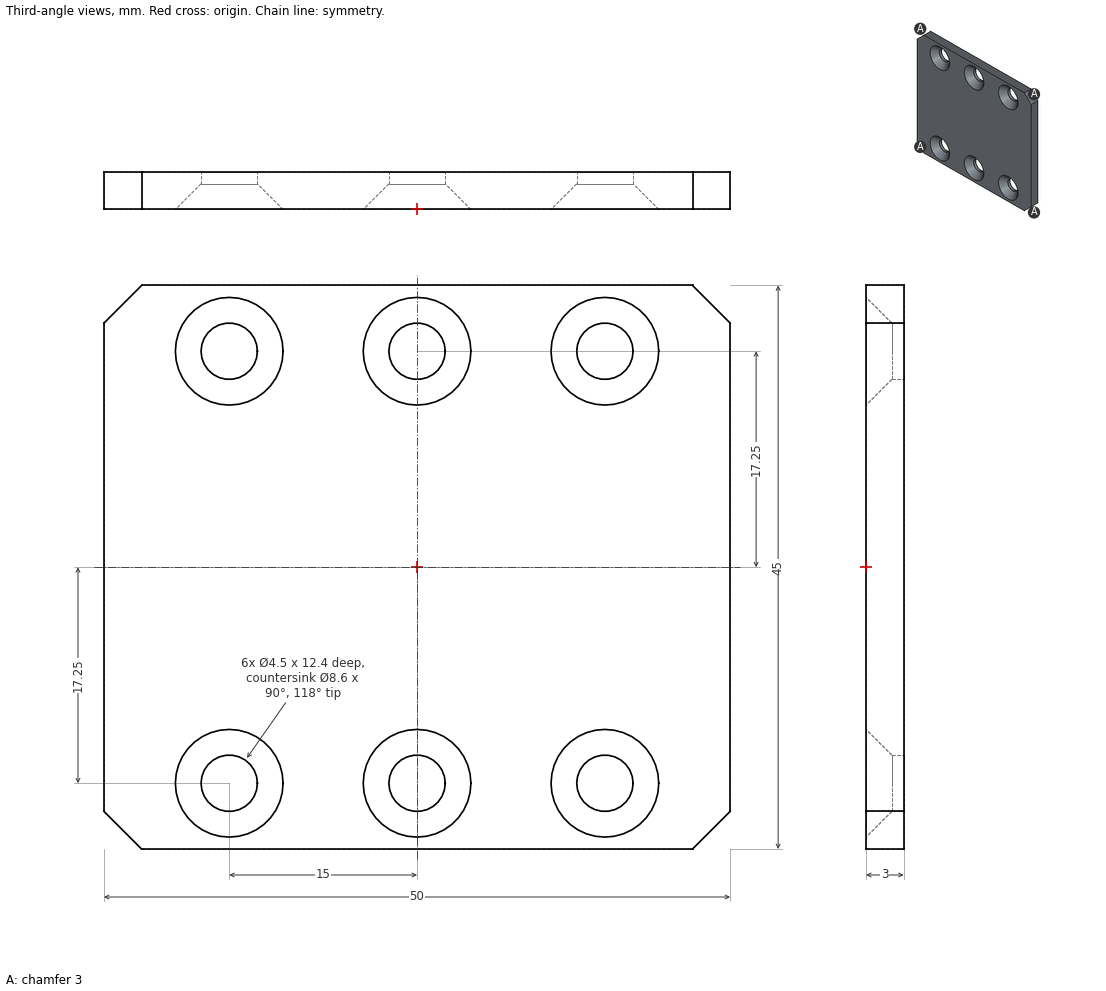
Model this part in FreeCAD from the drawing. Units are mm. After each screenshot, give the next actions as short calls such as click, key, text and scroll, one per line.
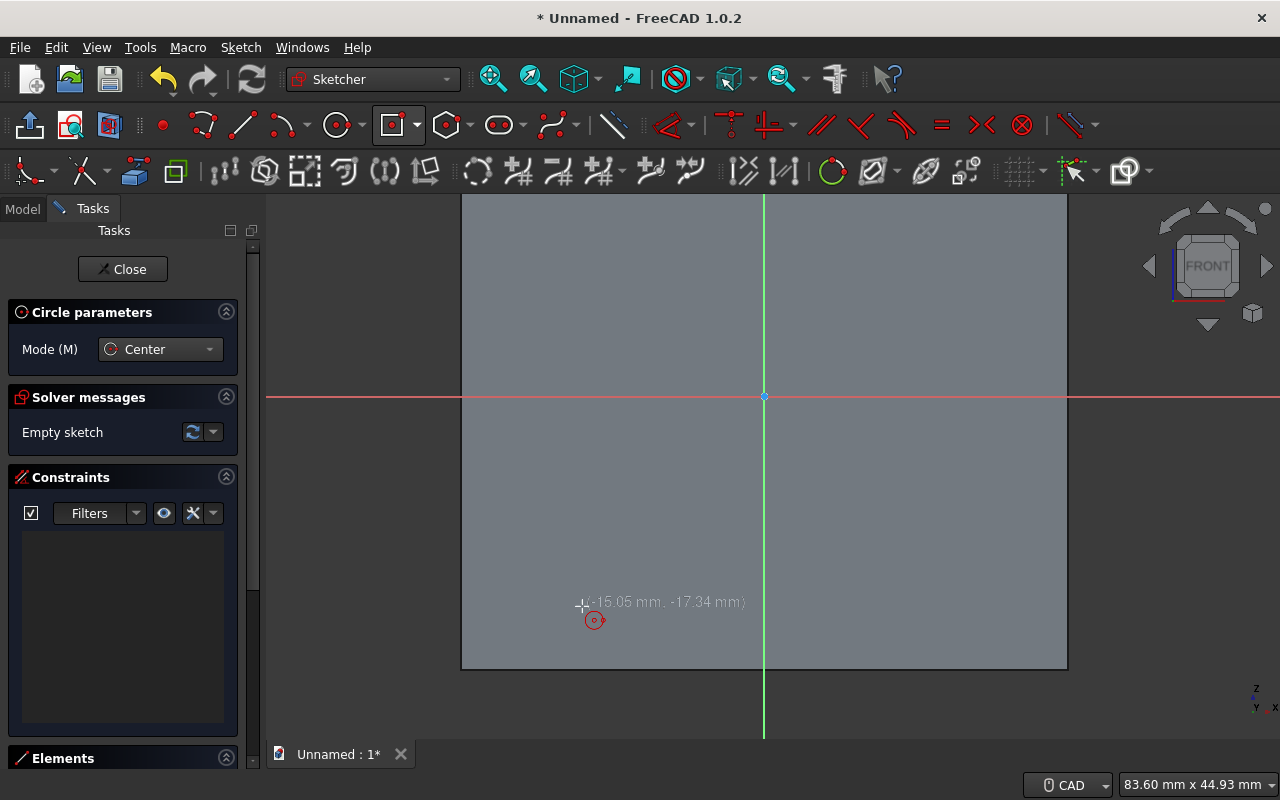
click(582, 606)
move(602, 587)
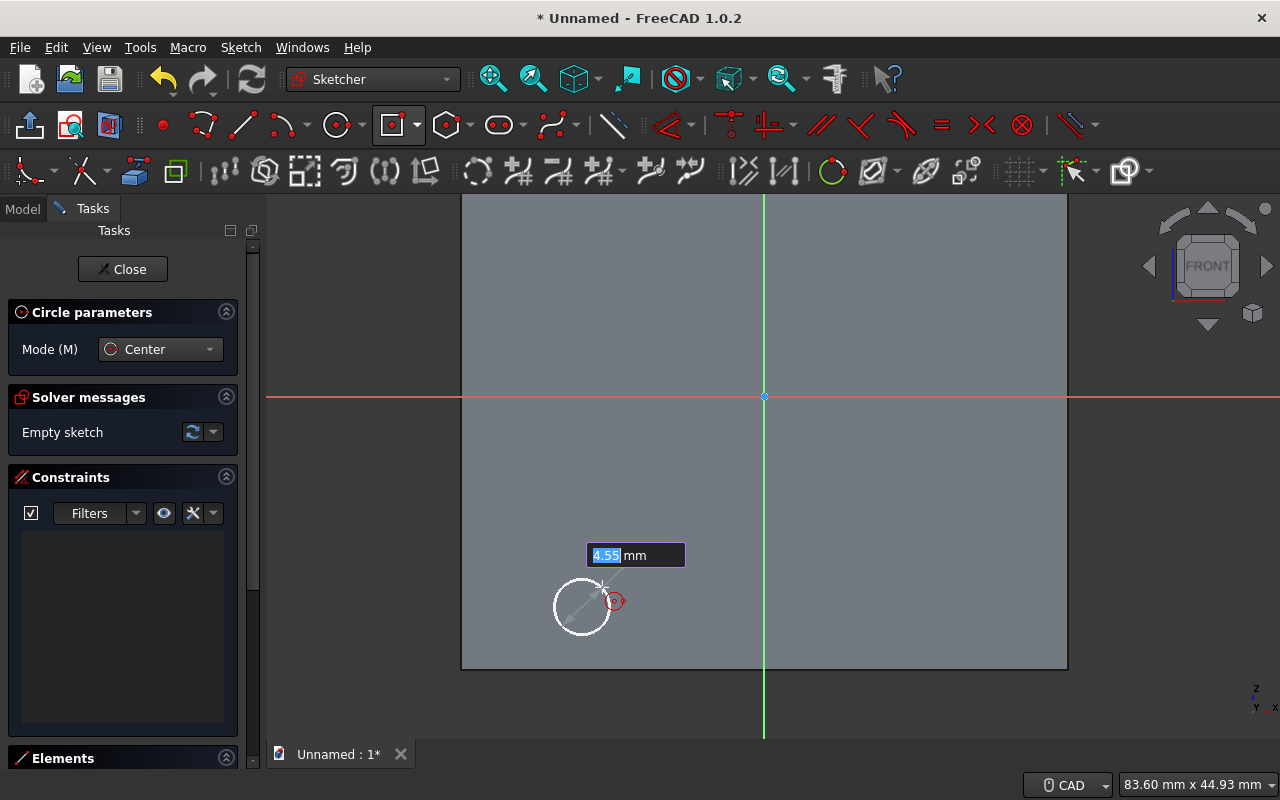
text(4.5)
key(Return)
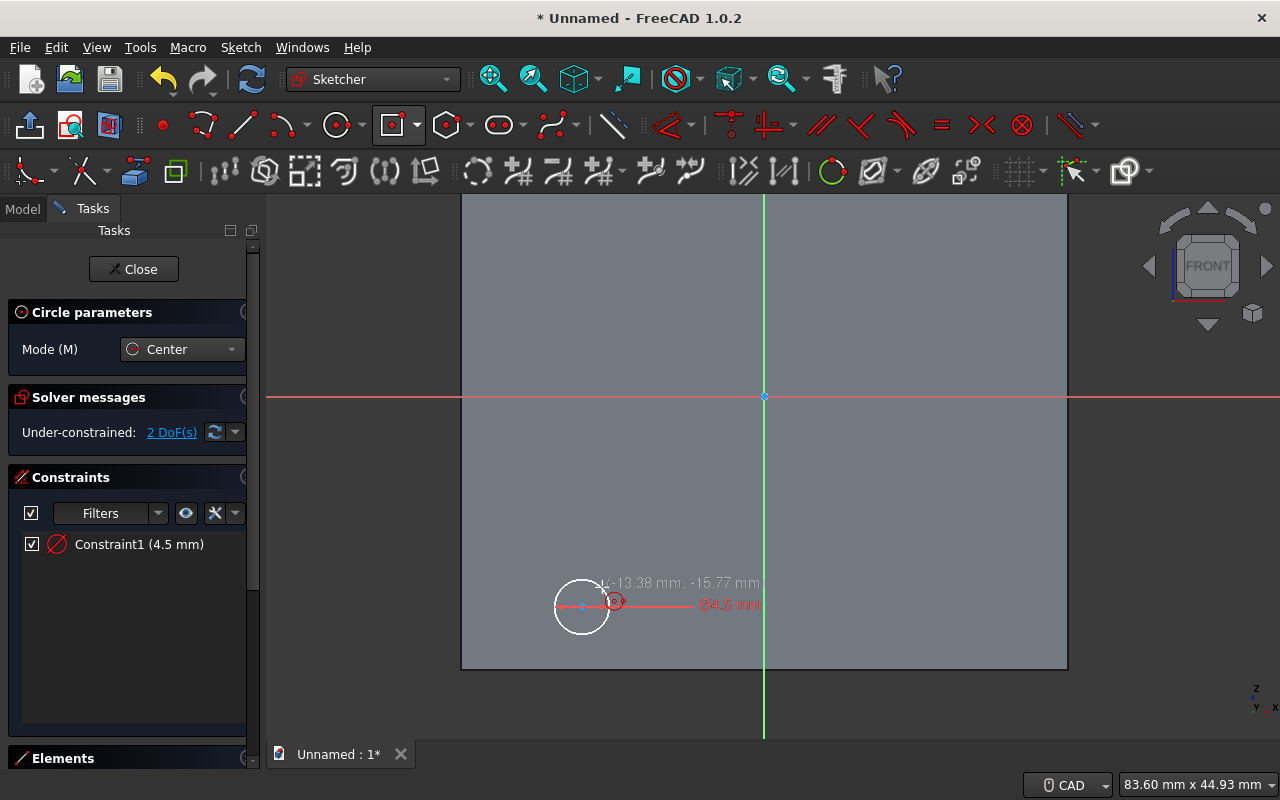
click(764, 606)
move(784, 587)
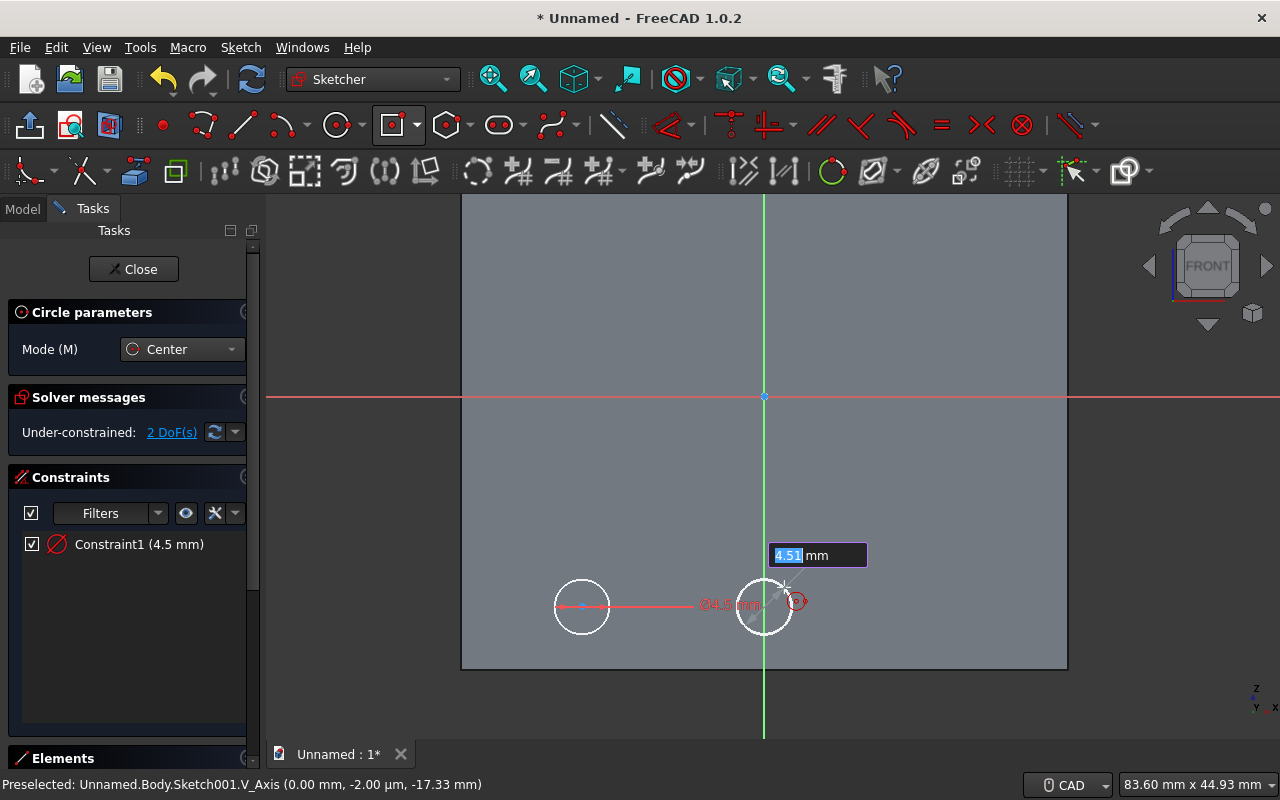
text(4.5)
key(Return)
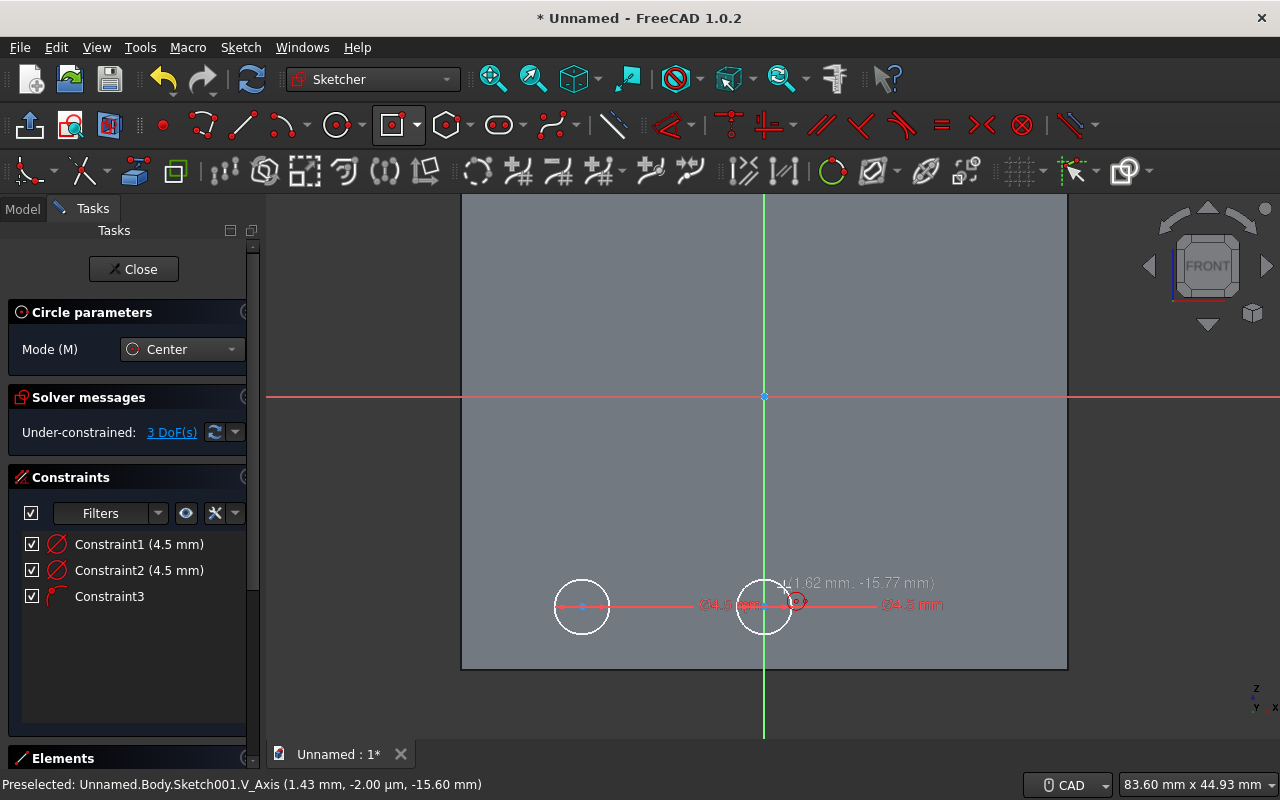
click(946, 606)
move(966, 587)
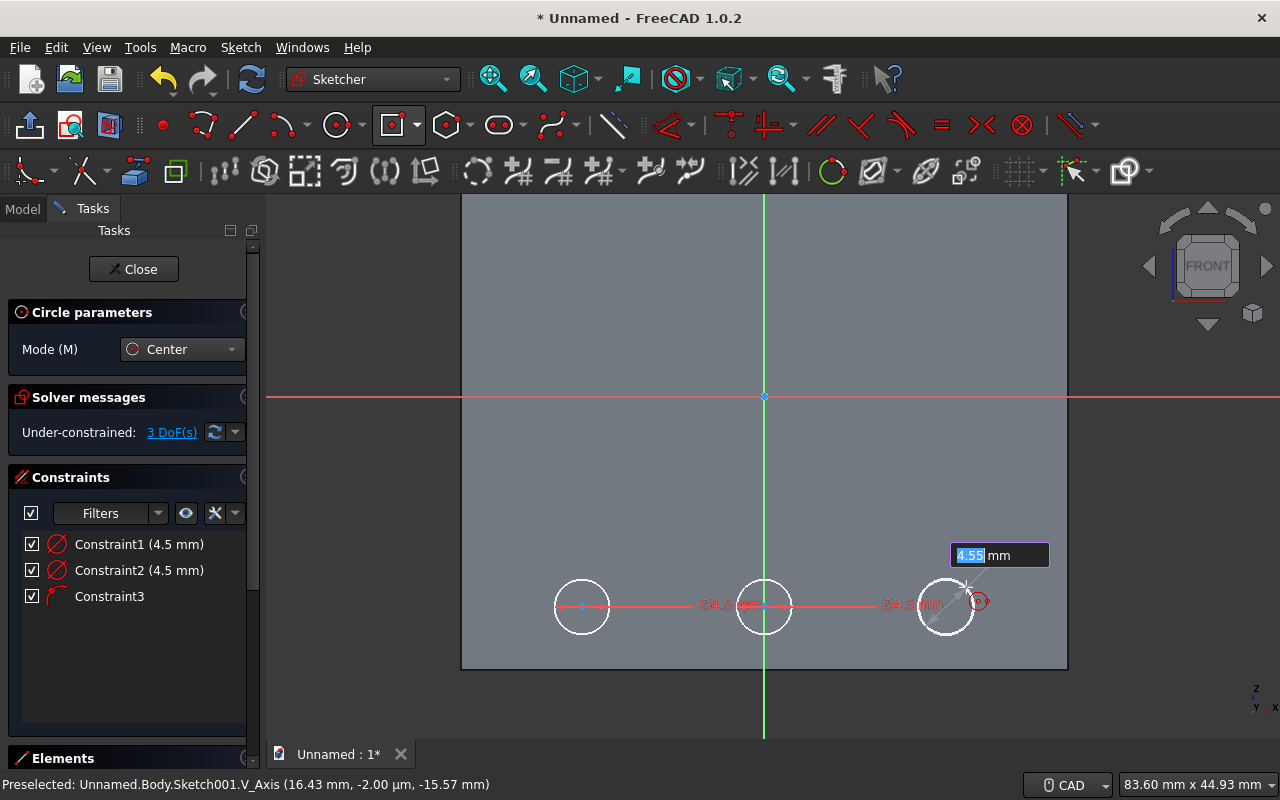
text(4.5)
key(Return)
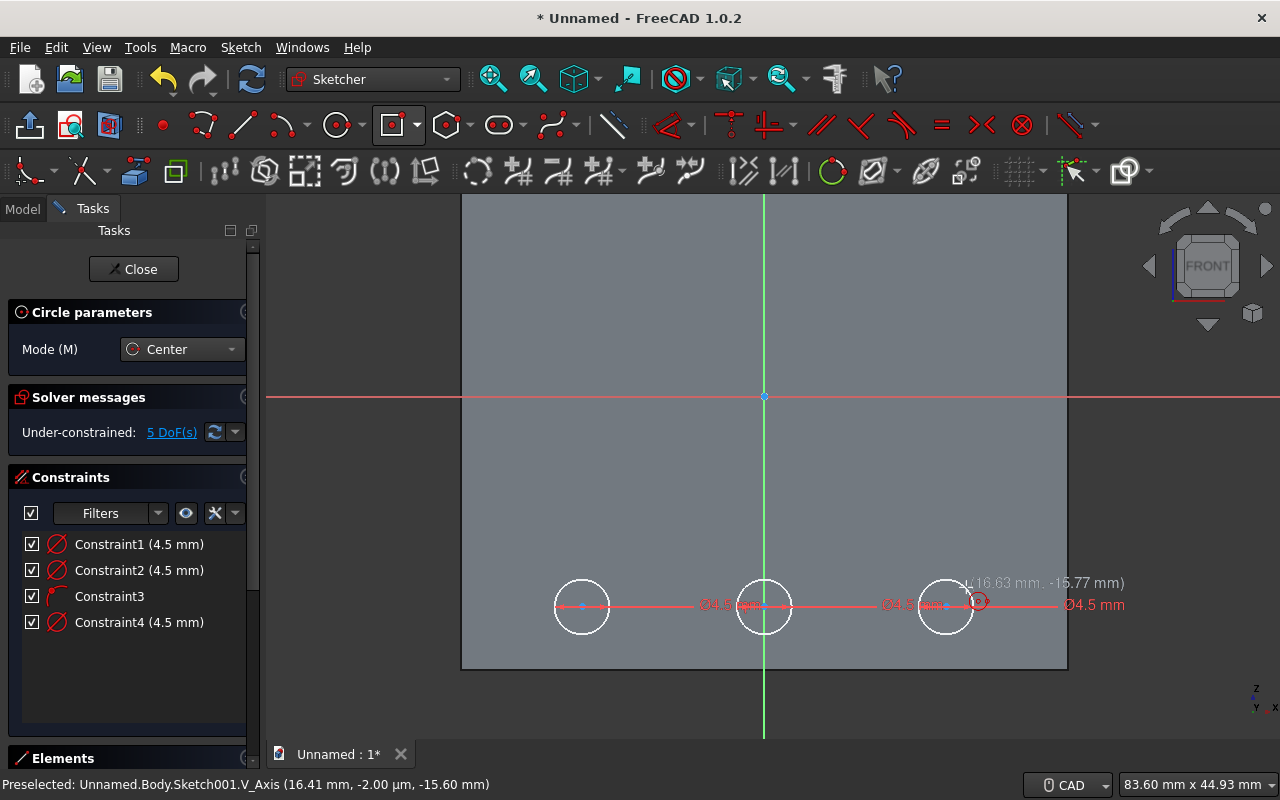
scroll(583, 608, down, 2)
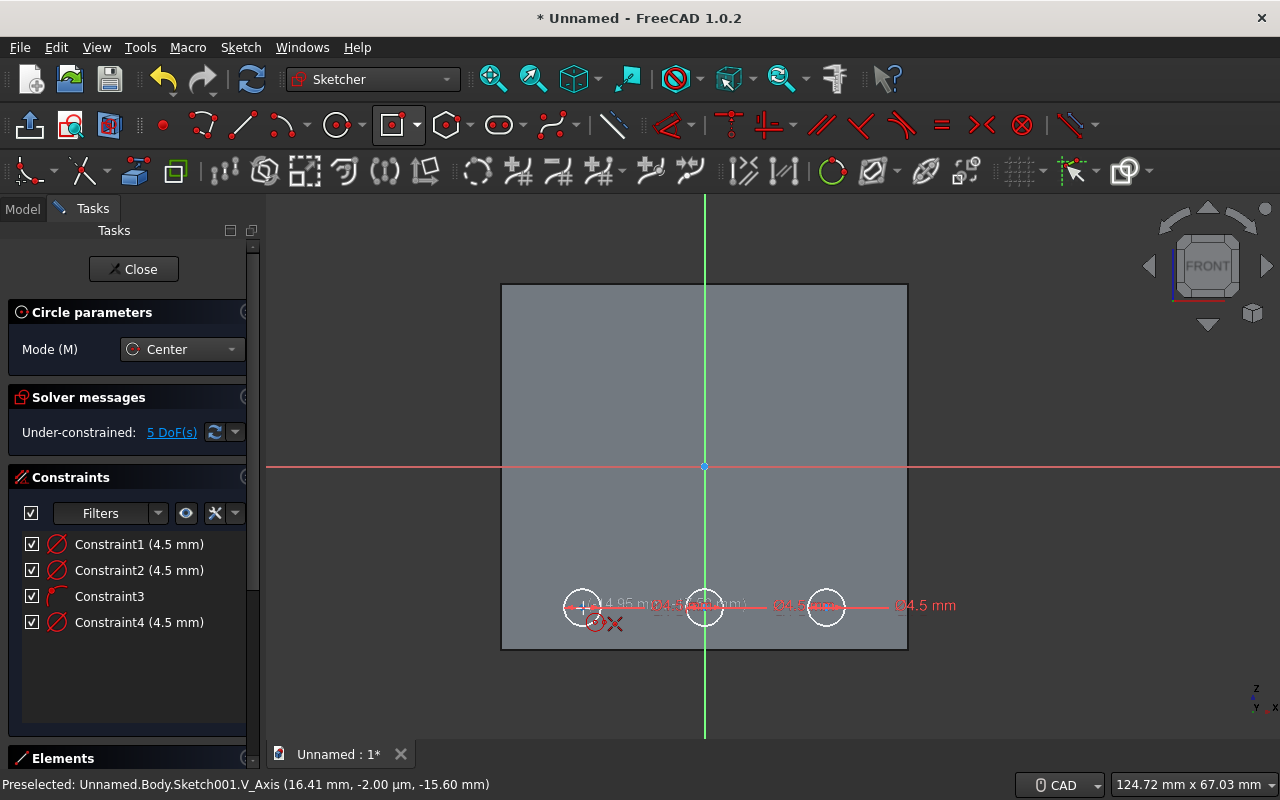
scroll(827, 326, up, 2)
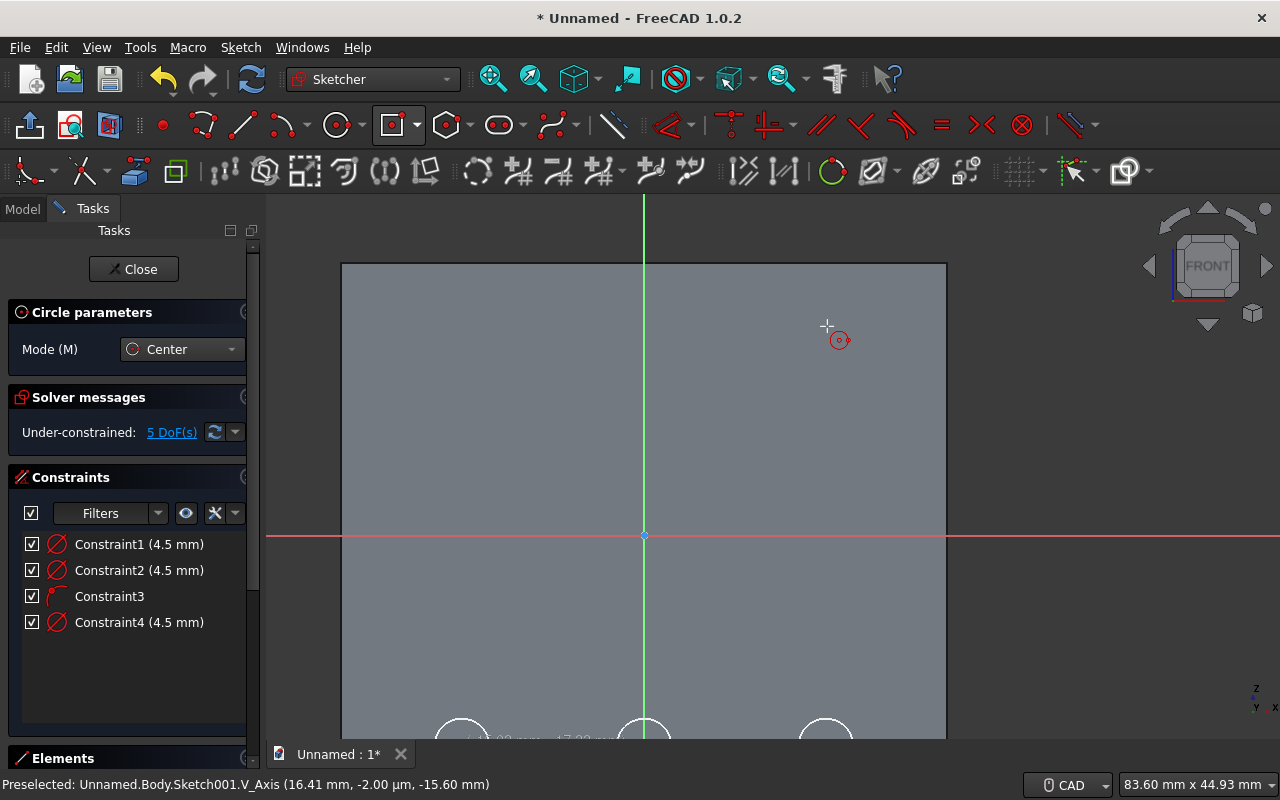
click(826, 327)
move(845, 307)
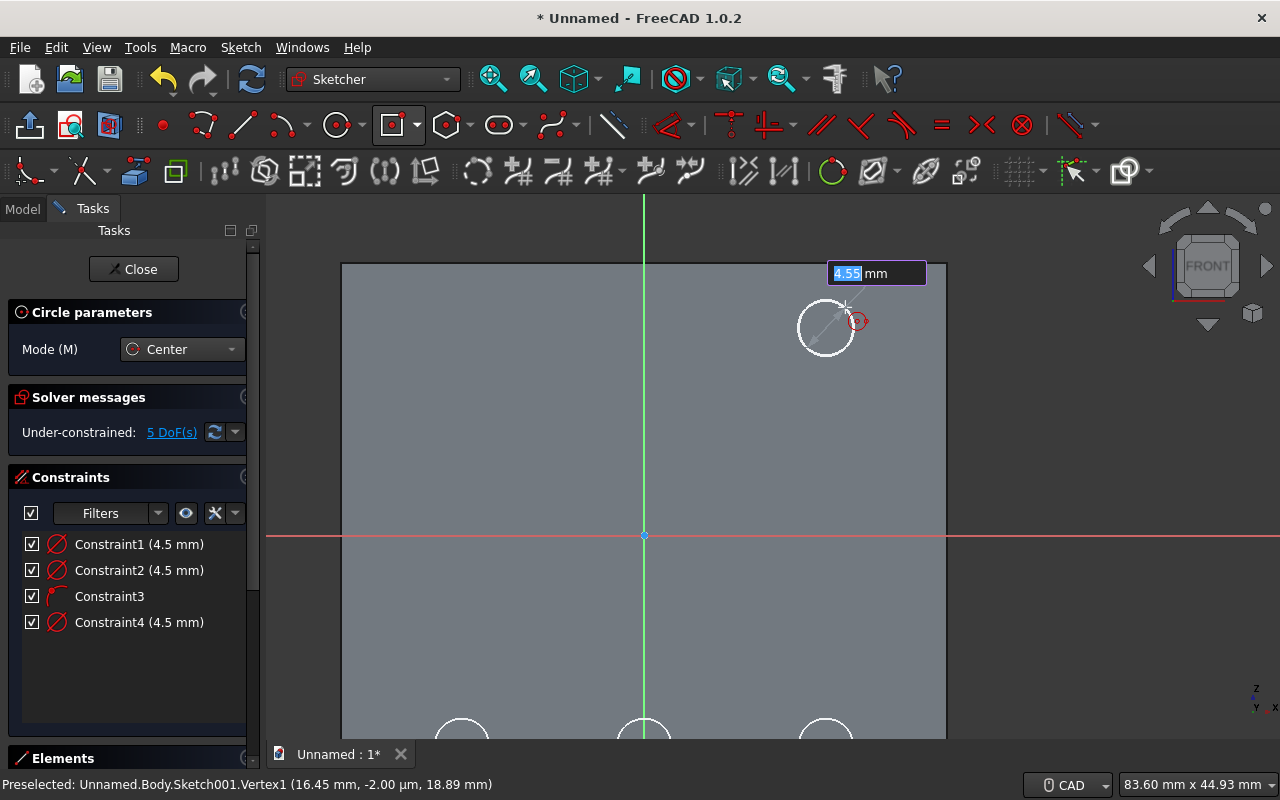
text(4.5)
key(Return)